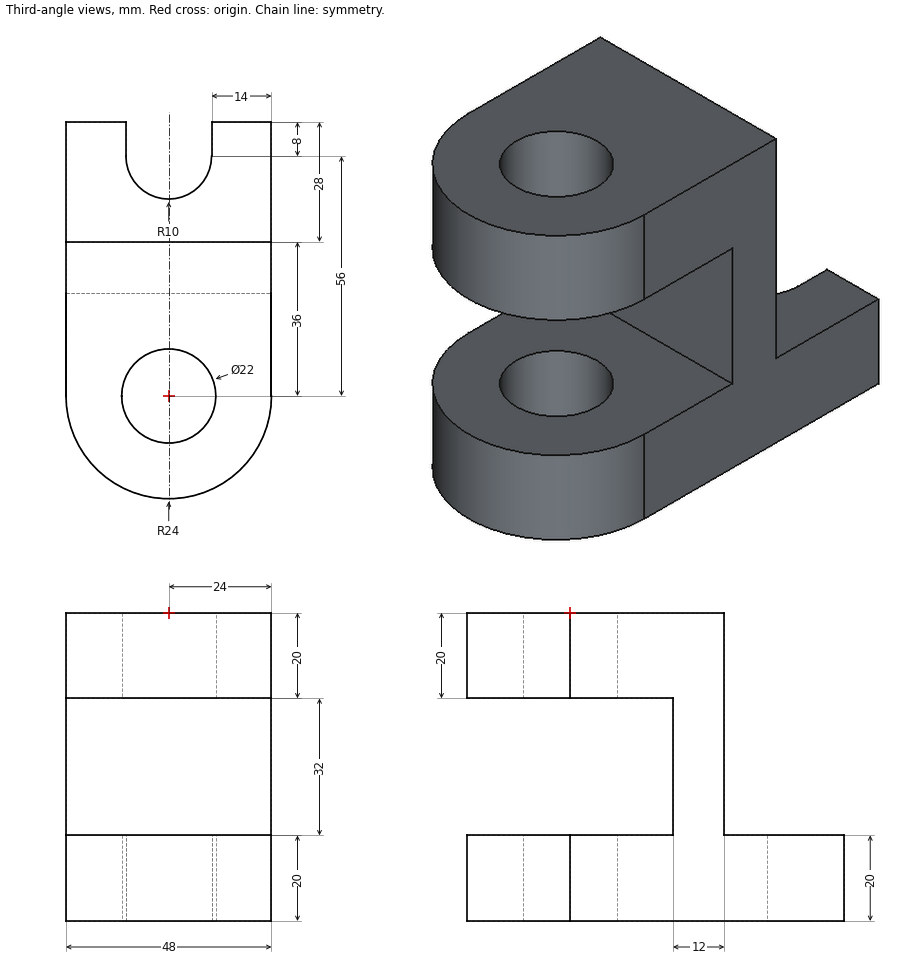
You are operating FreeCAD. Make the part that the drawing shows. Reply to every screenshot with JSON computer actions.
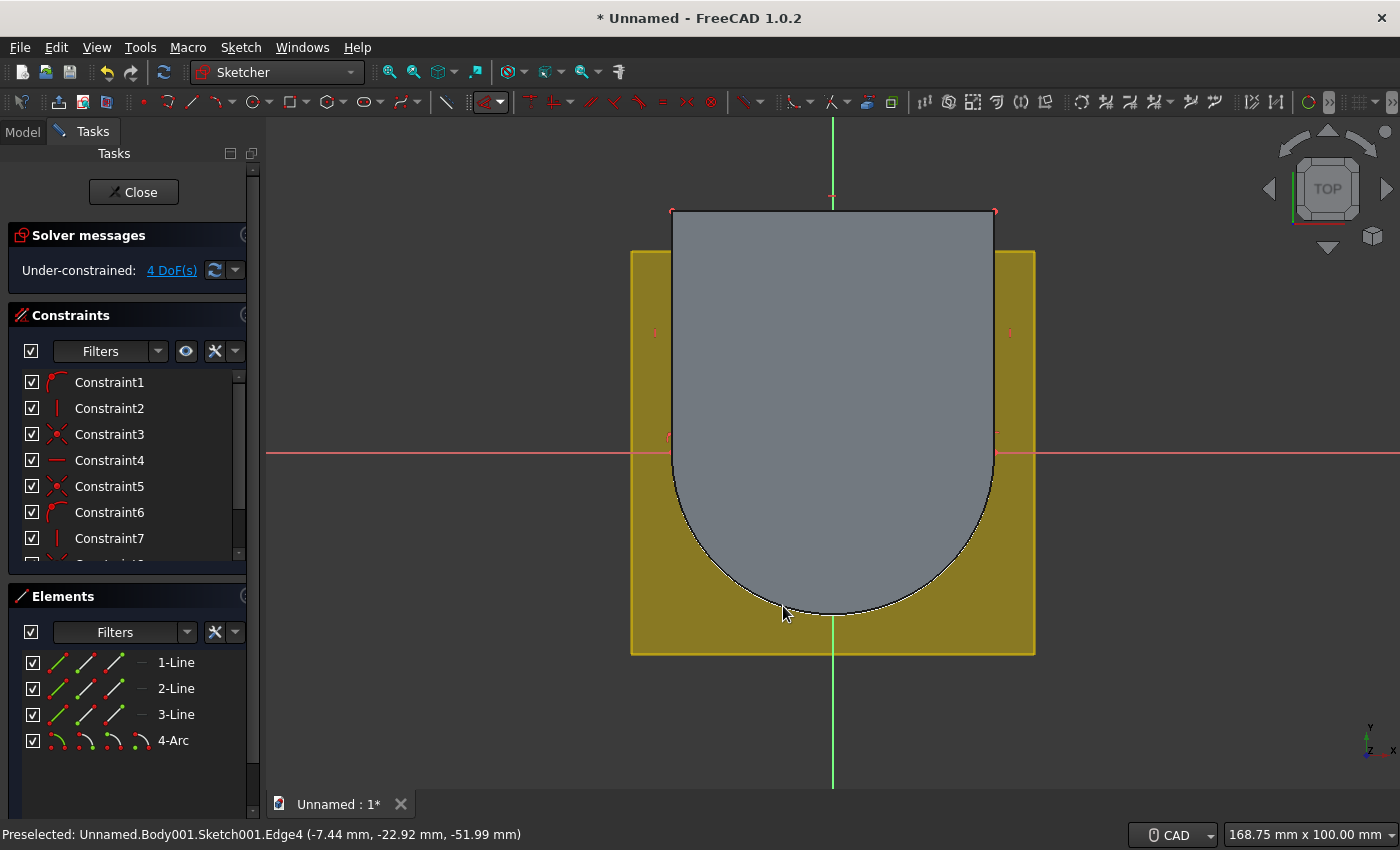
{"action": "left_click", "coordinate": [672, 381]}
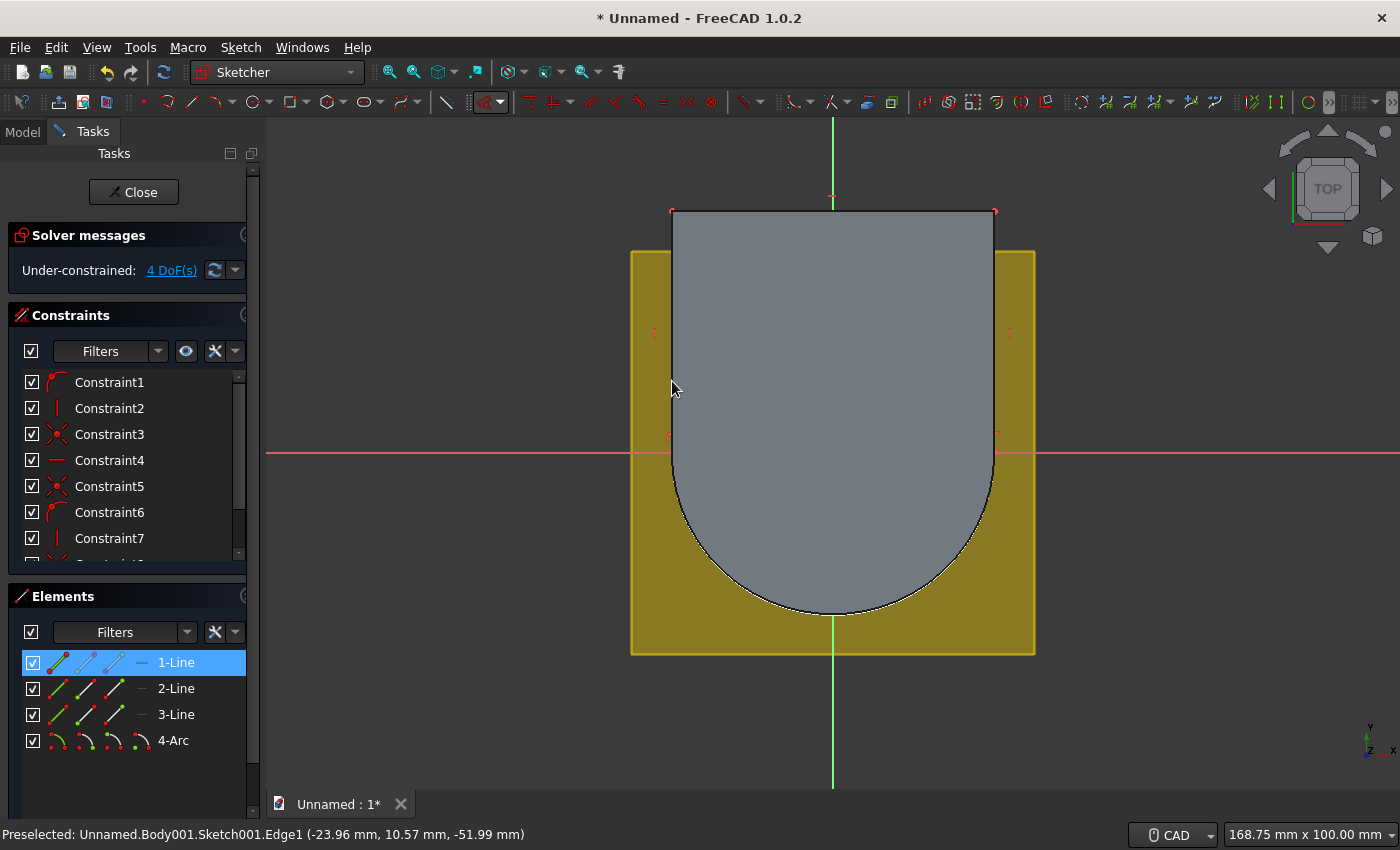
{"action": "left_click", "coordinate": [738, 584]}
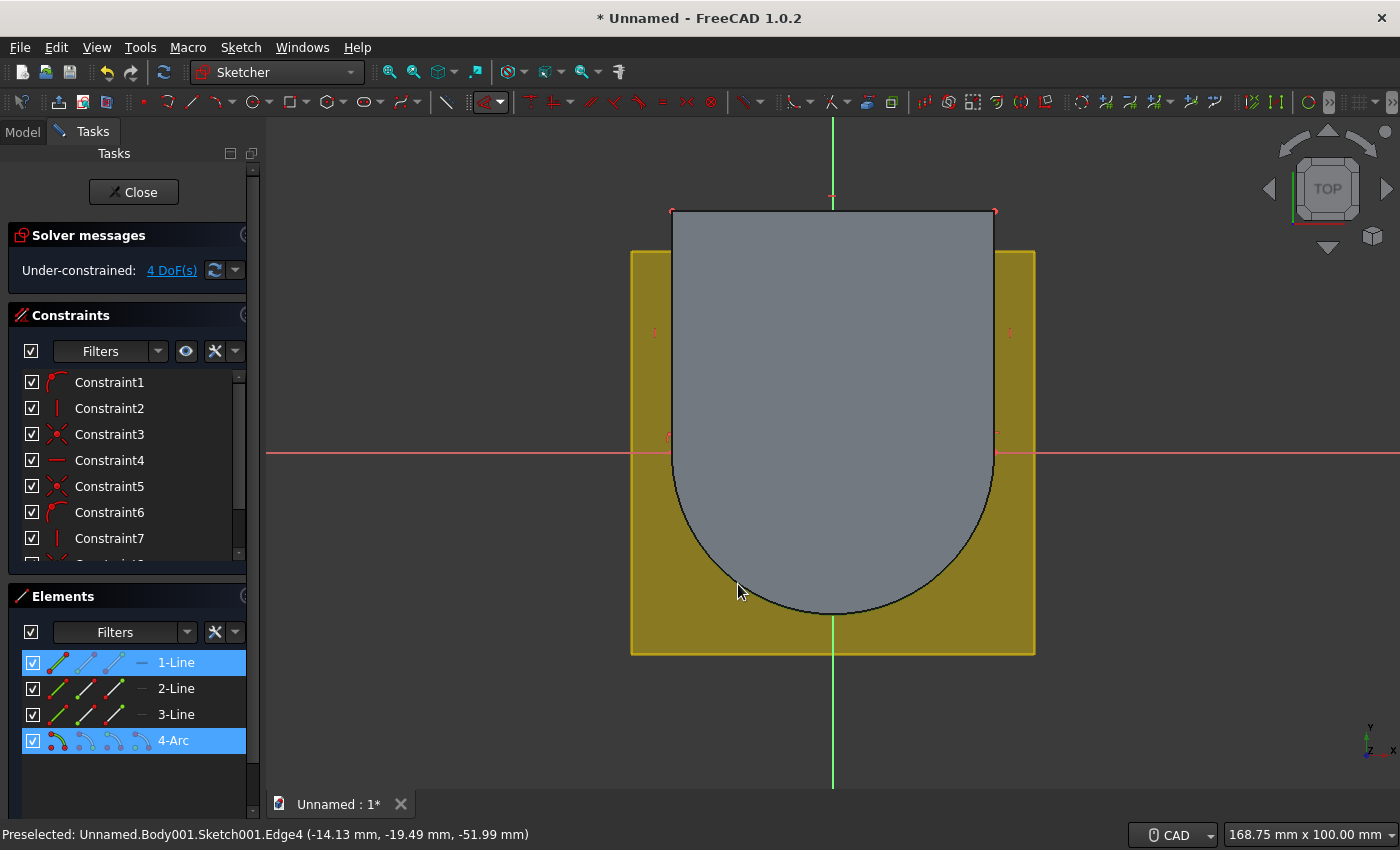
{"action": "left_click", "coordinate": [640, 102]}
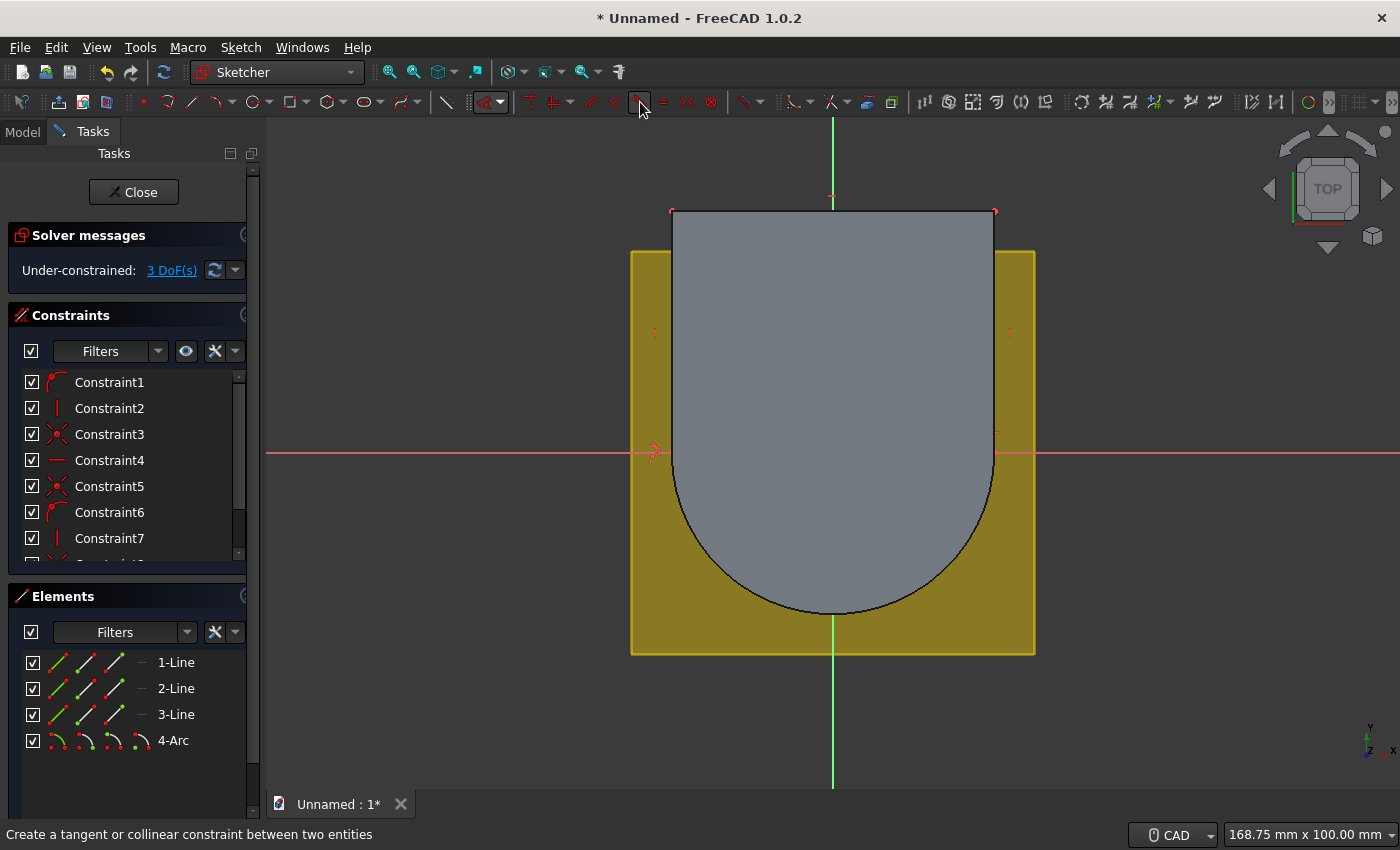
{"action": "left_click", "coordinate": [833, 453]}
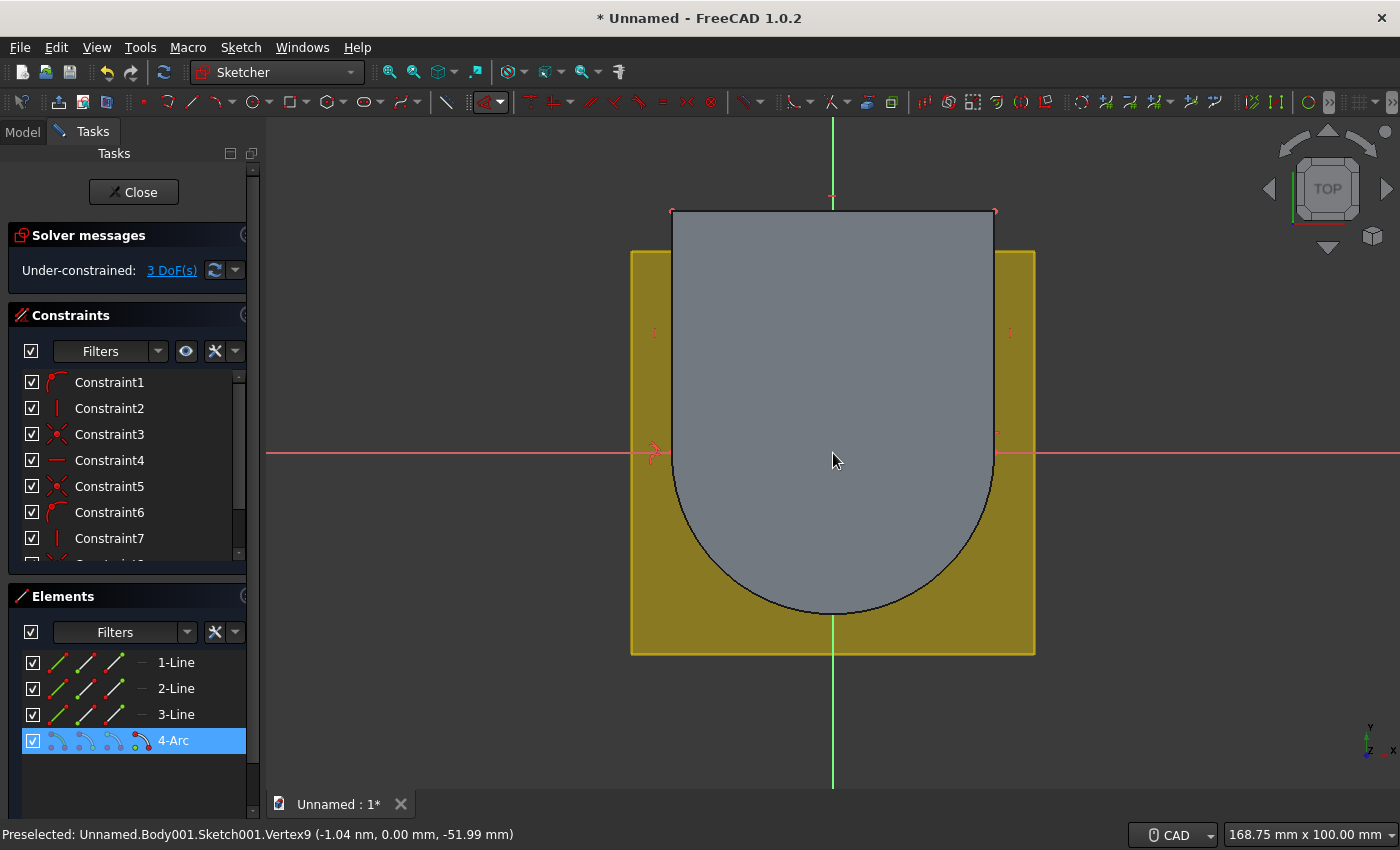
{"action": "left_click", "coordinate": [833, 717]}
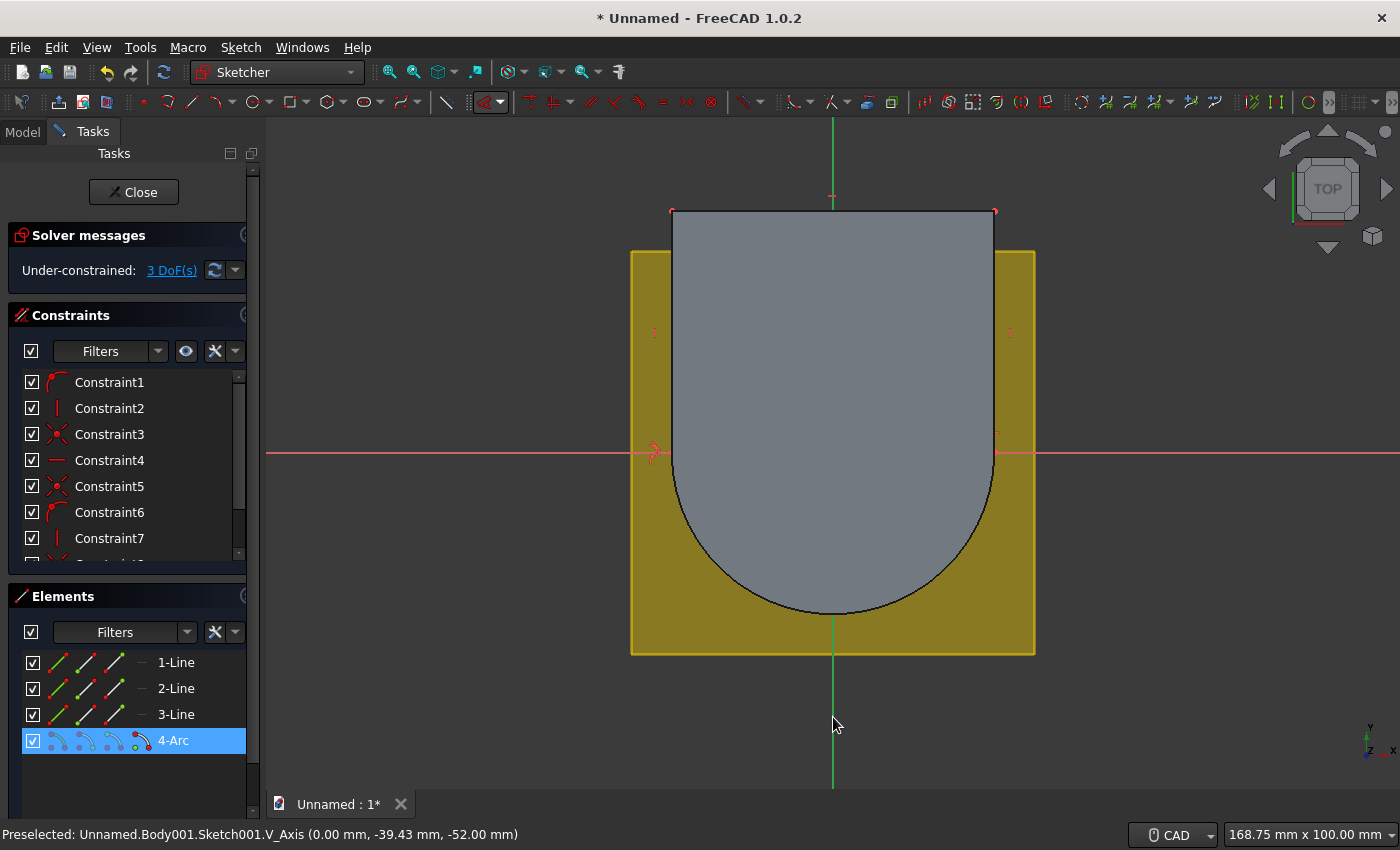
{"action": "left_click", "coordinate": [530, 102]}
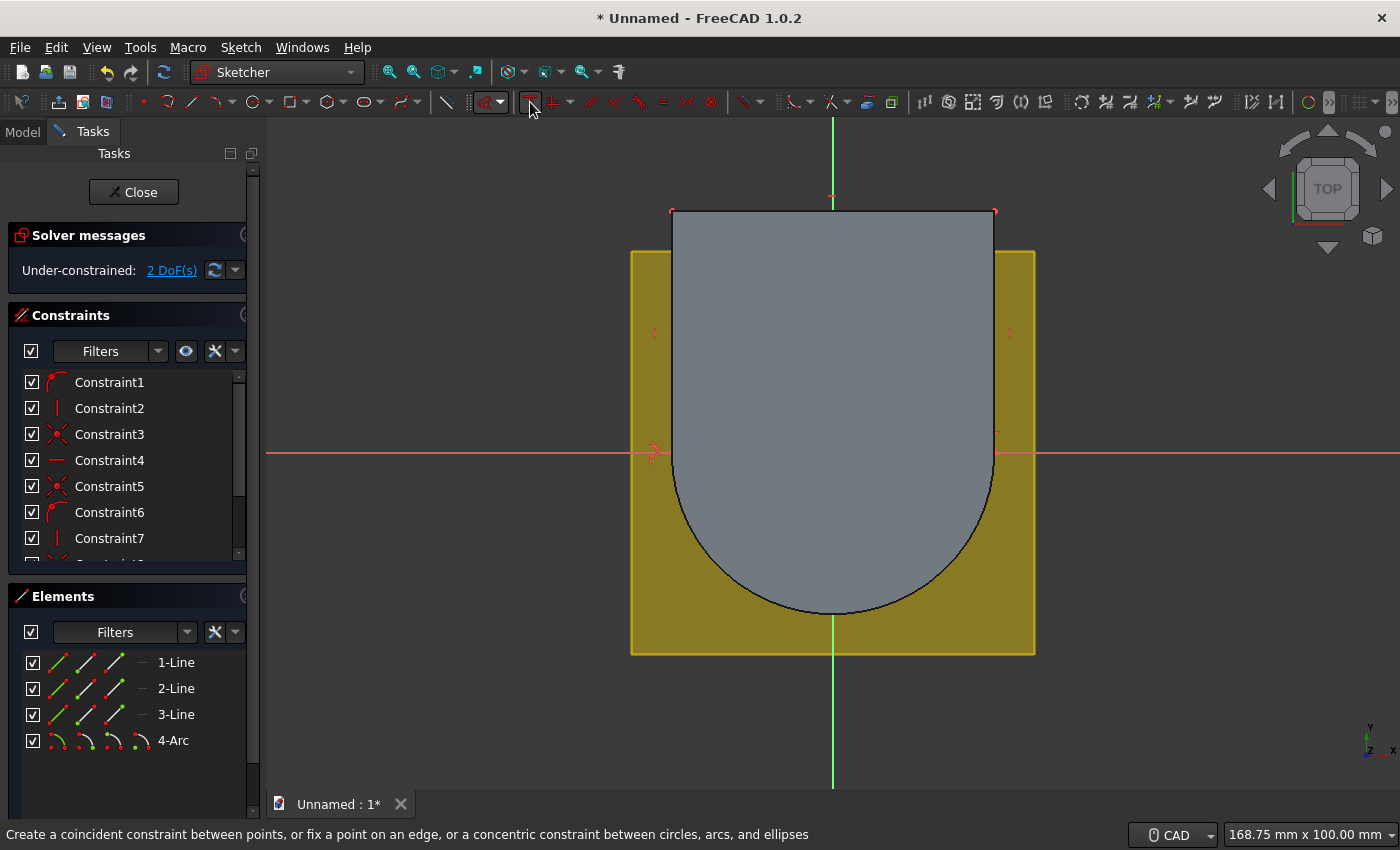
{"action": "left_click", "coordinate": [738, 583]}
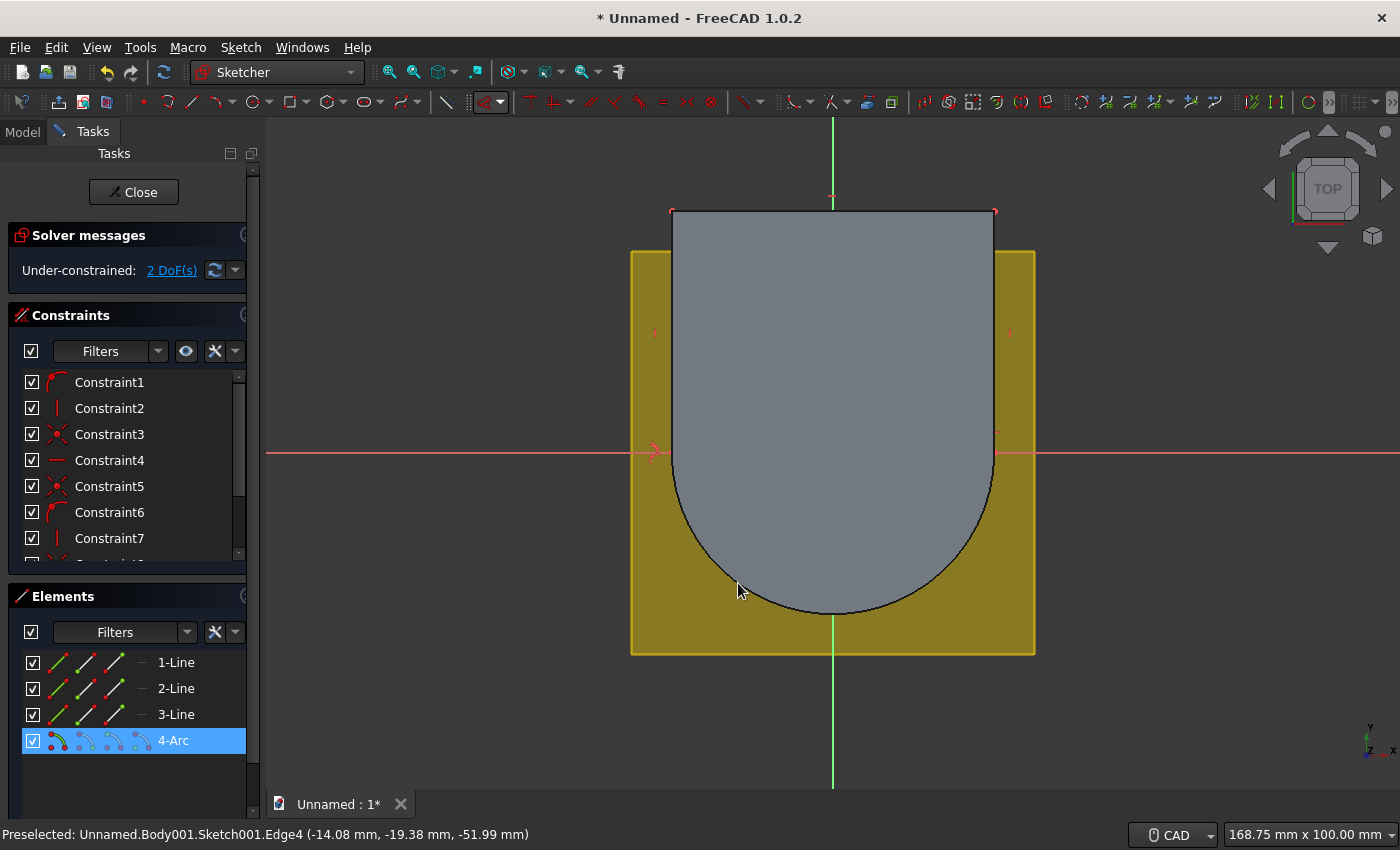
{"action": "key", "text": "k r"}